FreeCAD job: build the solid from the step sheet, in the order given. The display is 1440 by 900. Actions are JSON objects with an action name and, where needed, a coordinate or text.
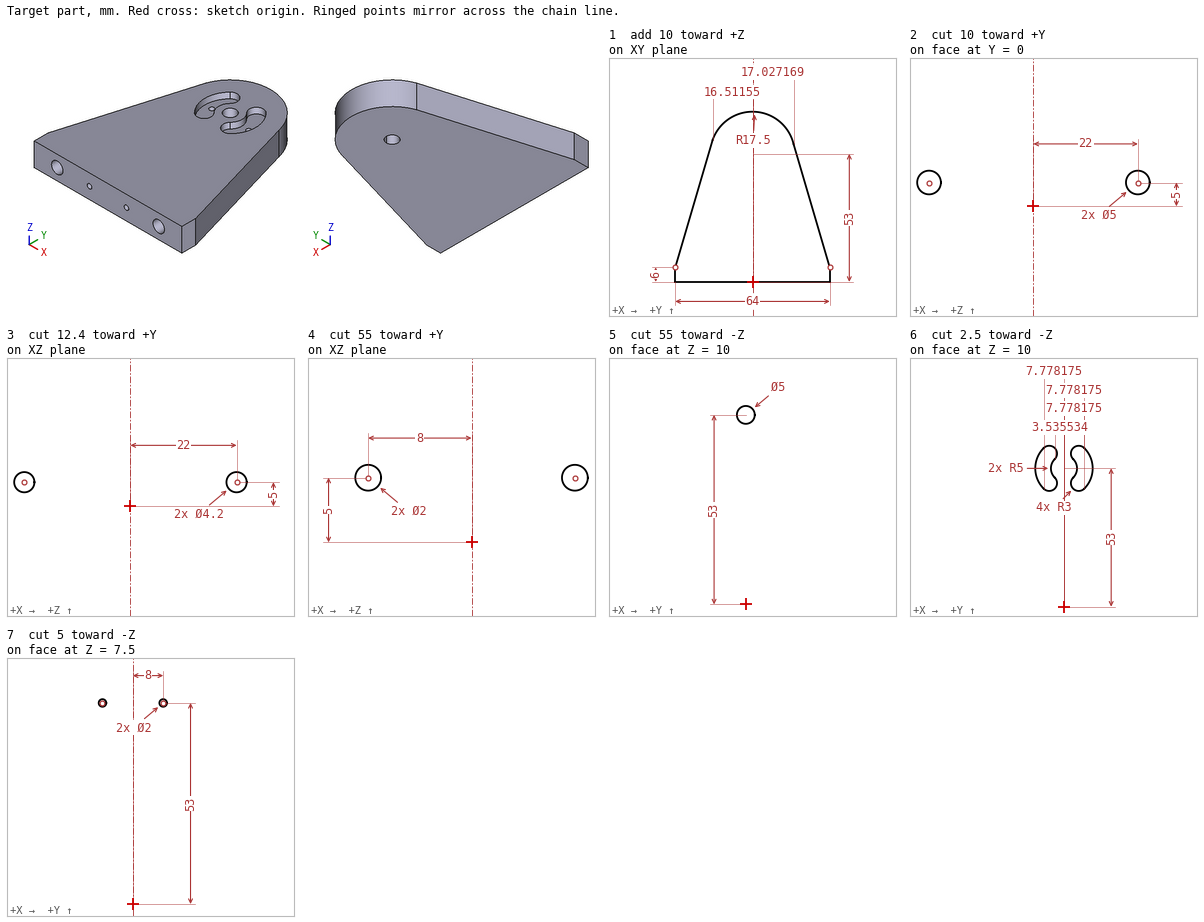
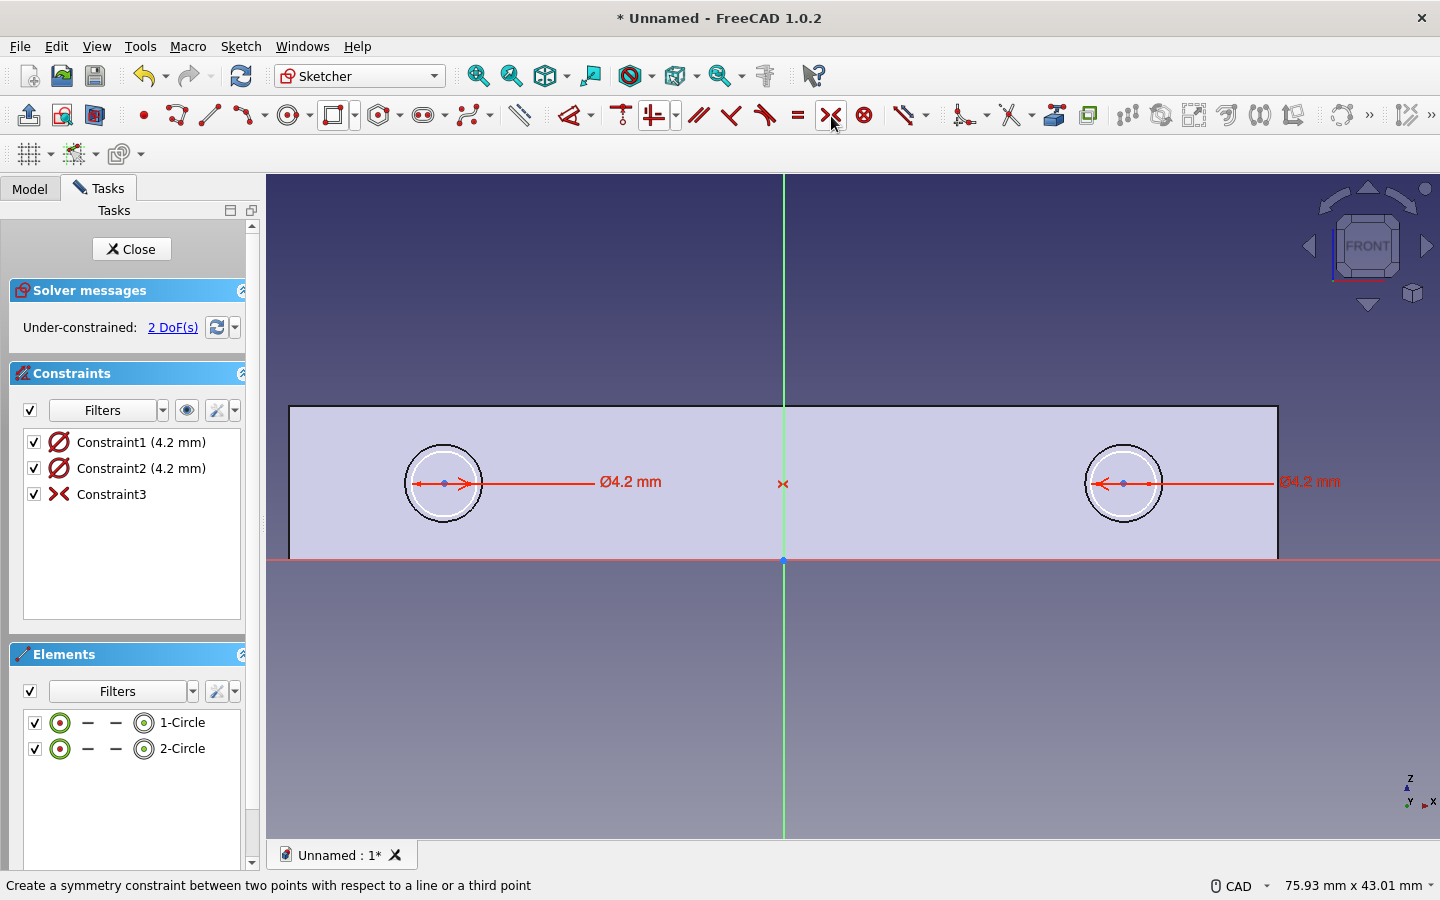
{"action": "left_click", "coordinate": [1123, 484]}
{"action": "left_click", "coordinate": [1157, 522]}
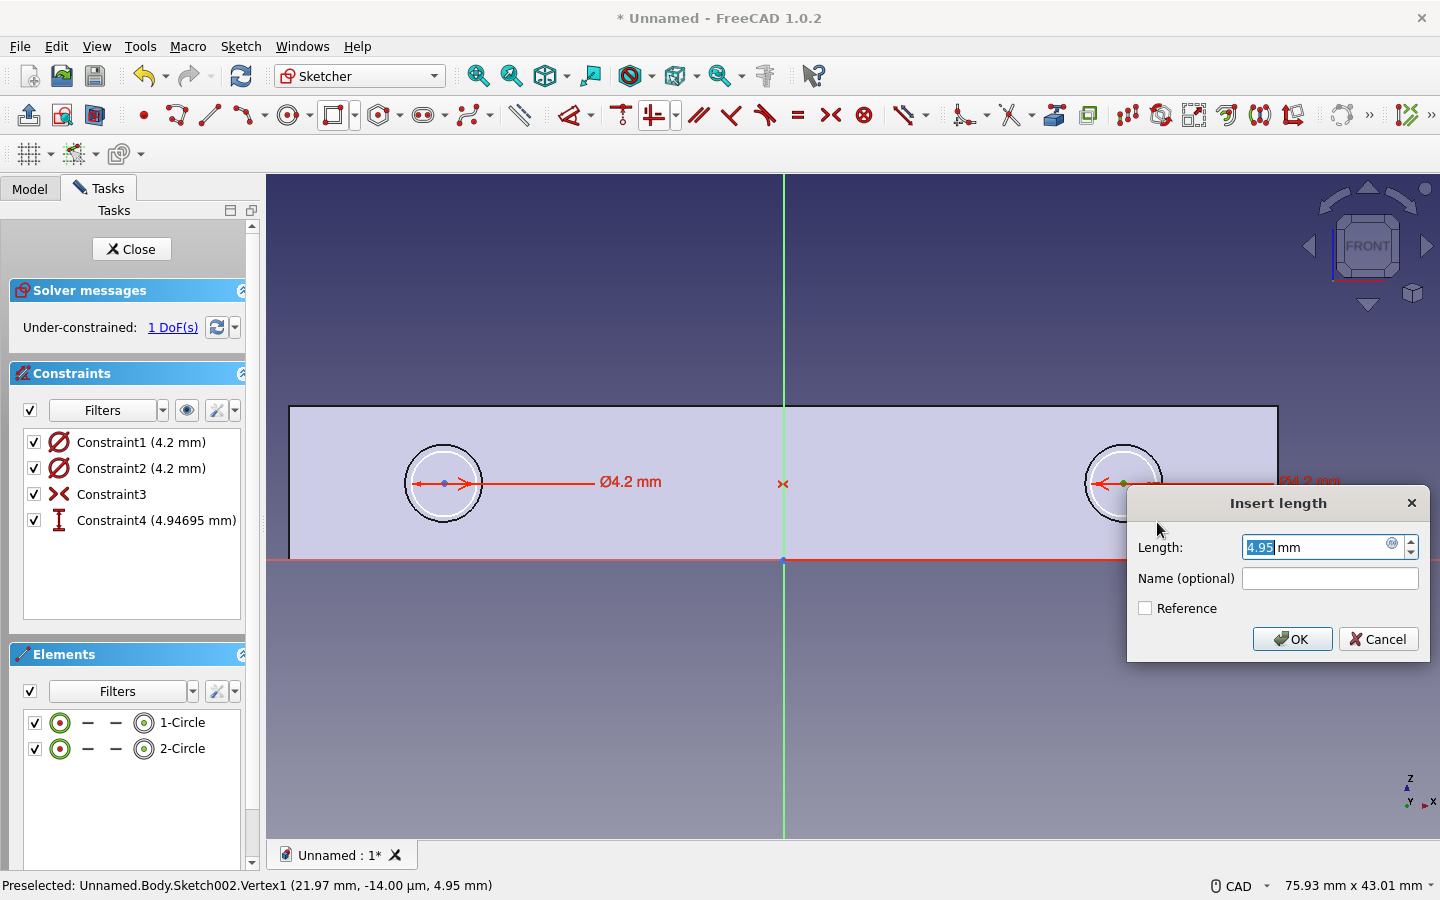
{"action": "type", "text": "5"}
{"action": "key", "text": "Return"}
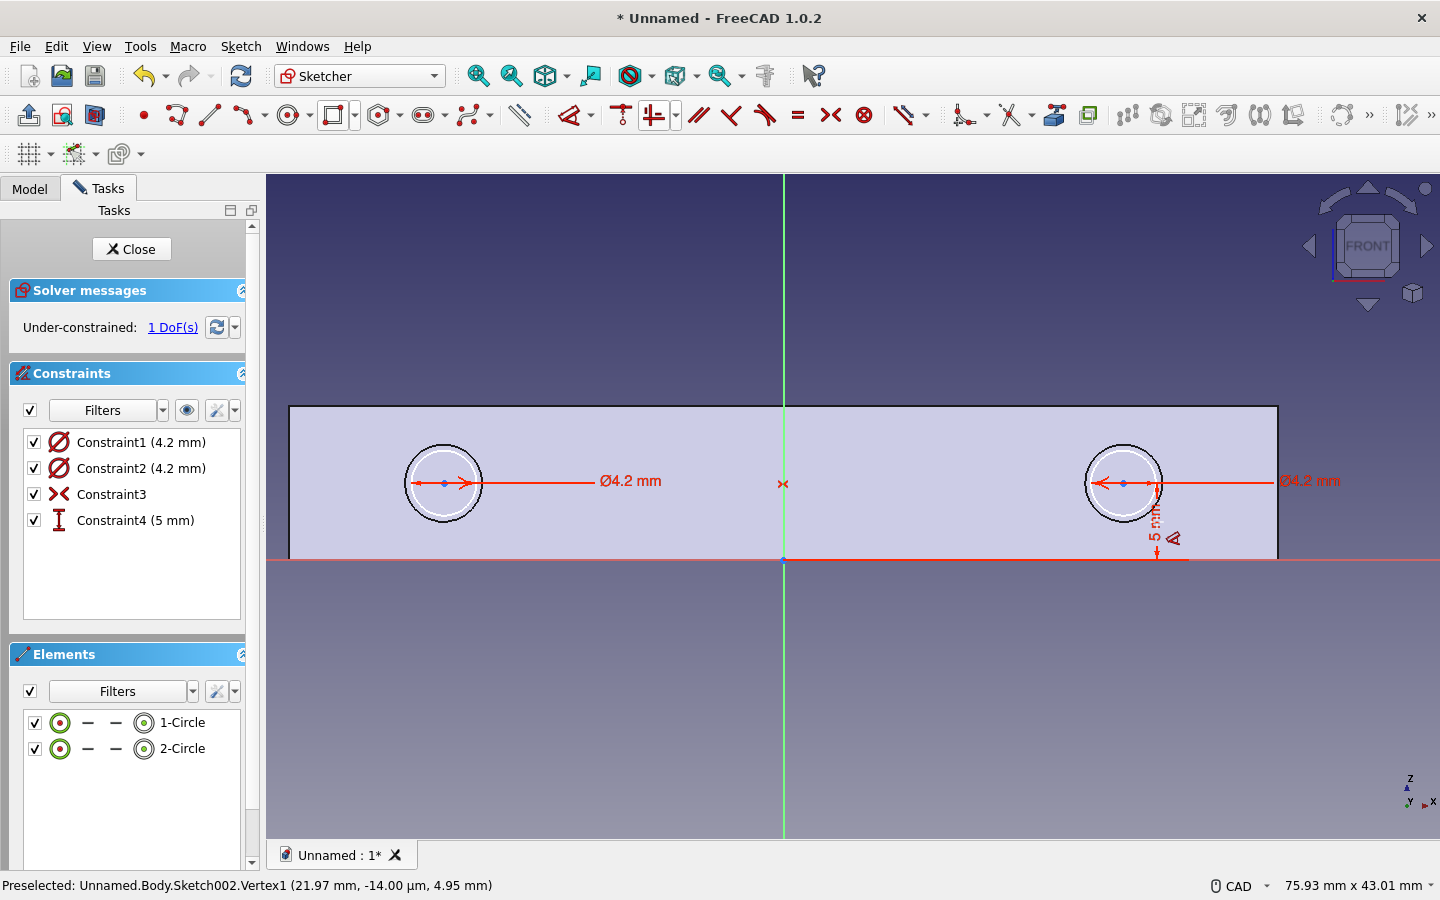
{"action": "left_click", "coordinate": [1123, 483]}
{"action": "left_click", "coordinate": [954, 594]}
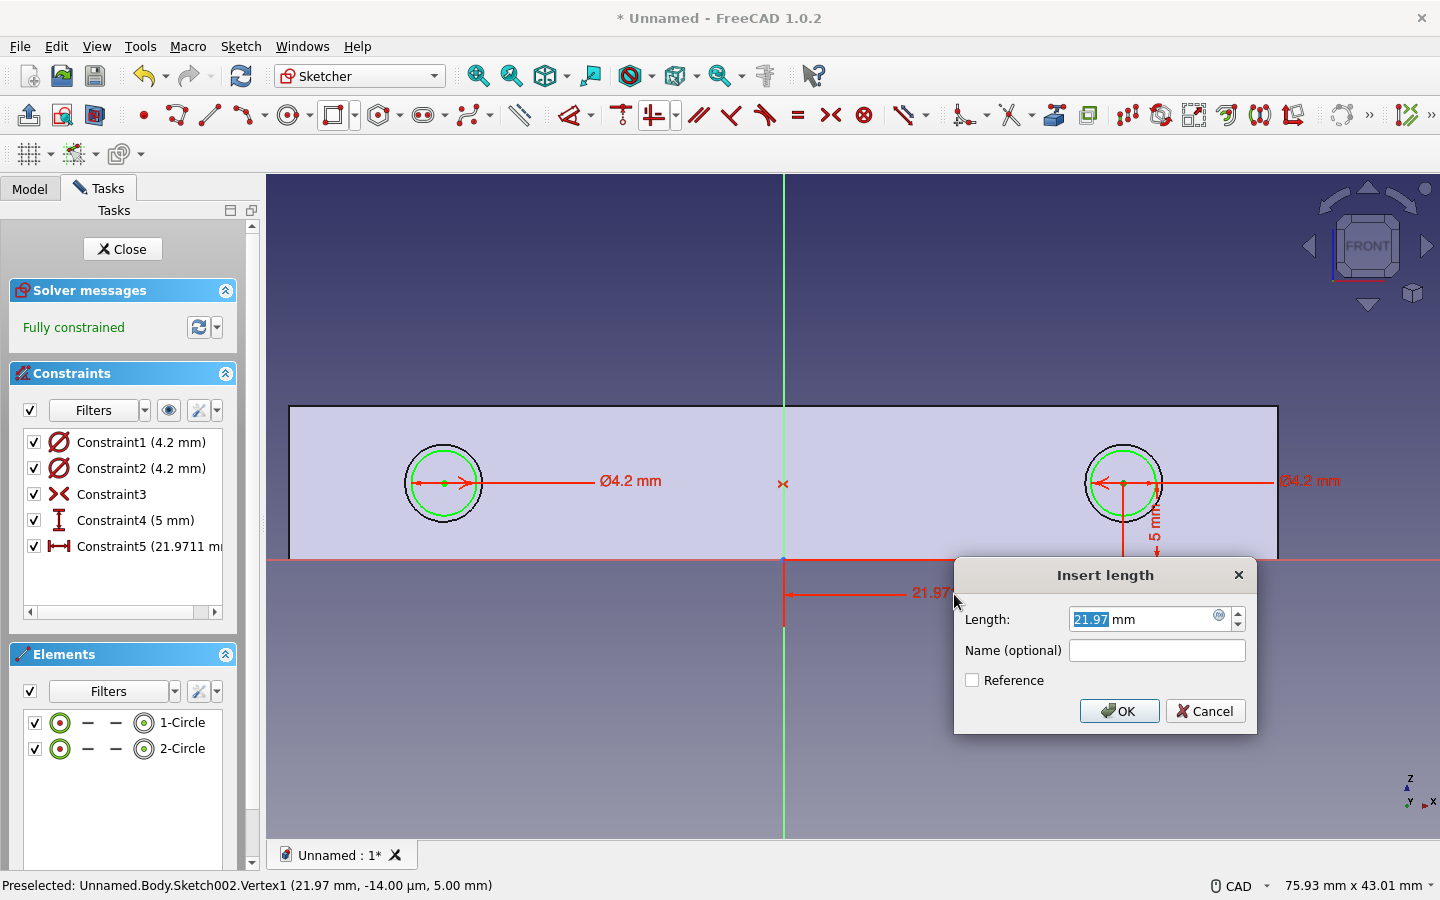
{"action": "type", "text": "22"}
{"action": "key", "text": "Return"}
{"action": "key", "text": "Escape"}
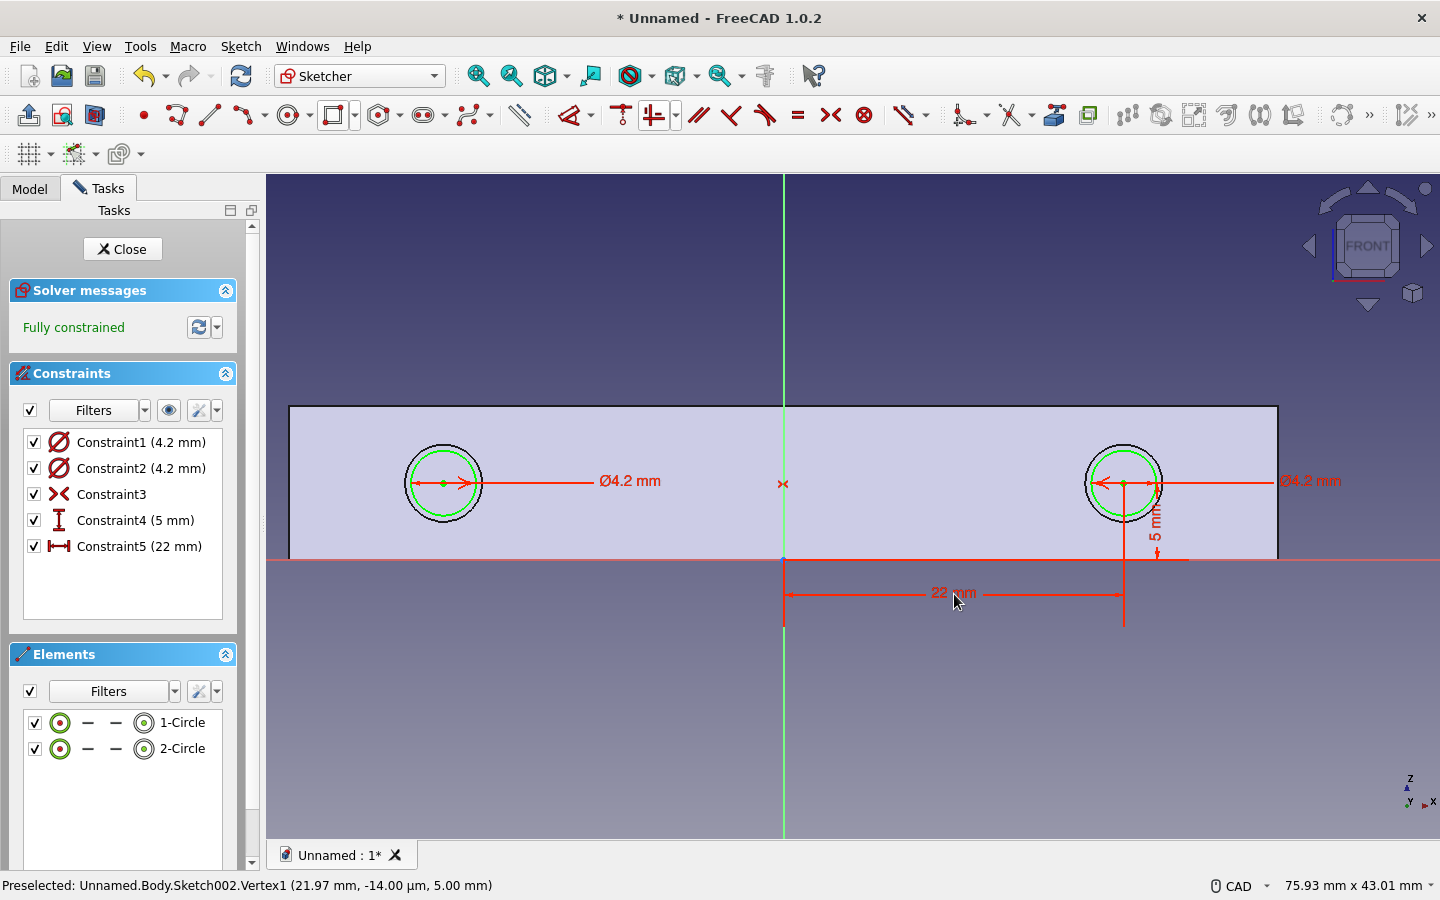
{"action": "left_click", "coordinate": [123, 249]}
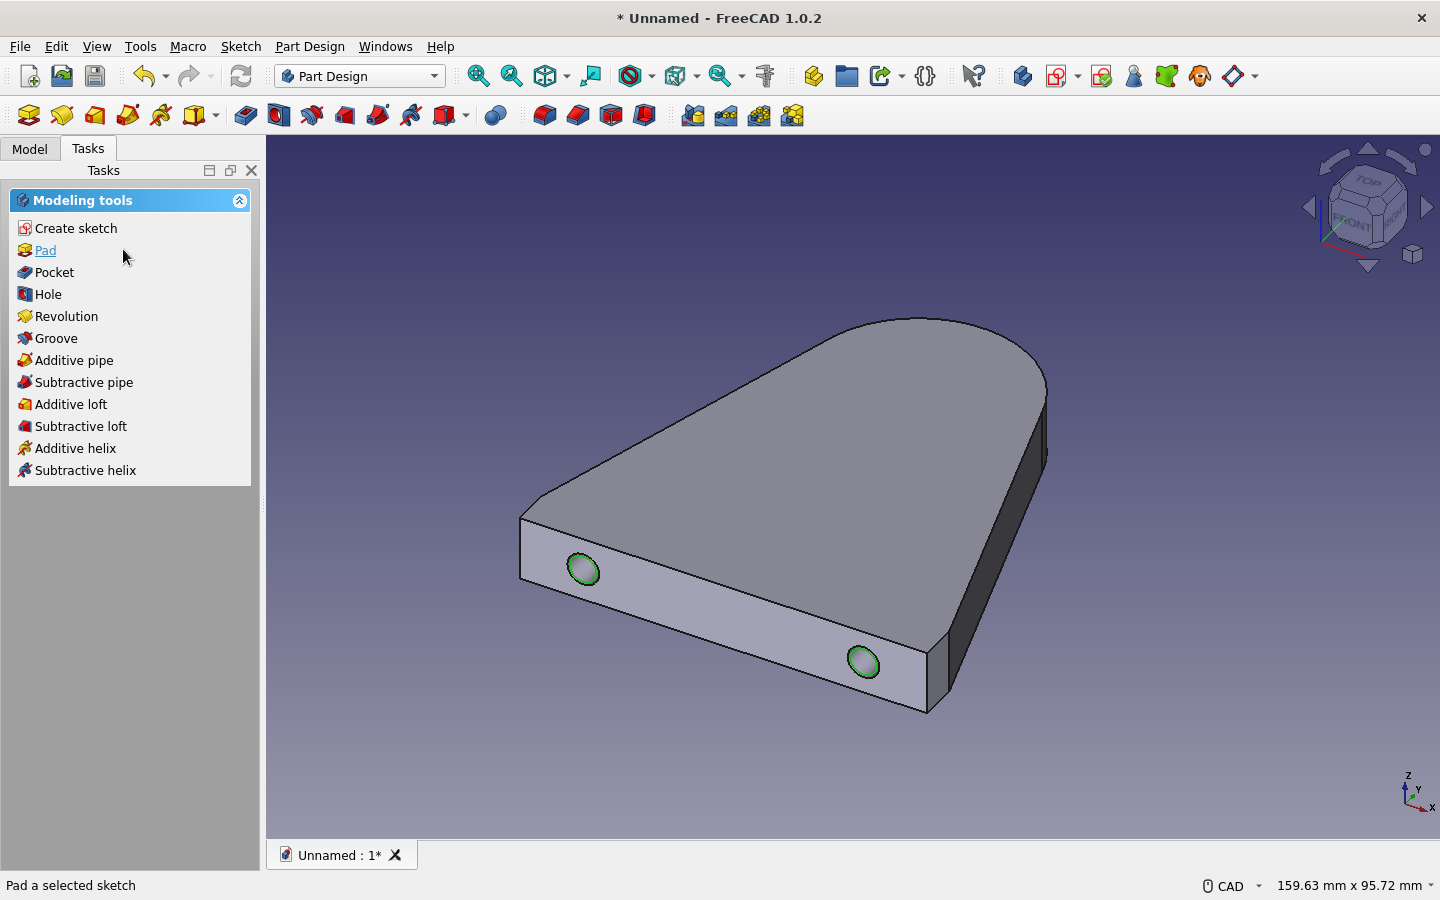
{"action": "left_click", "coordinate": [246, 116]}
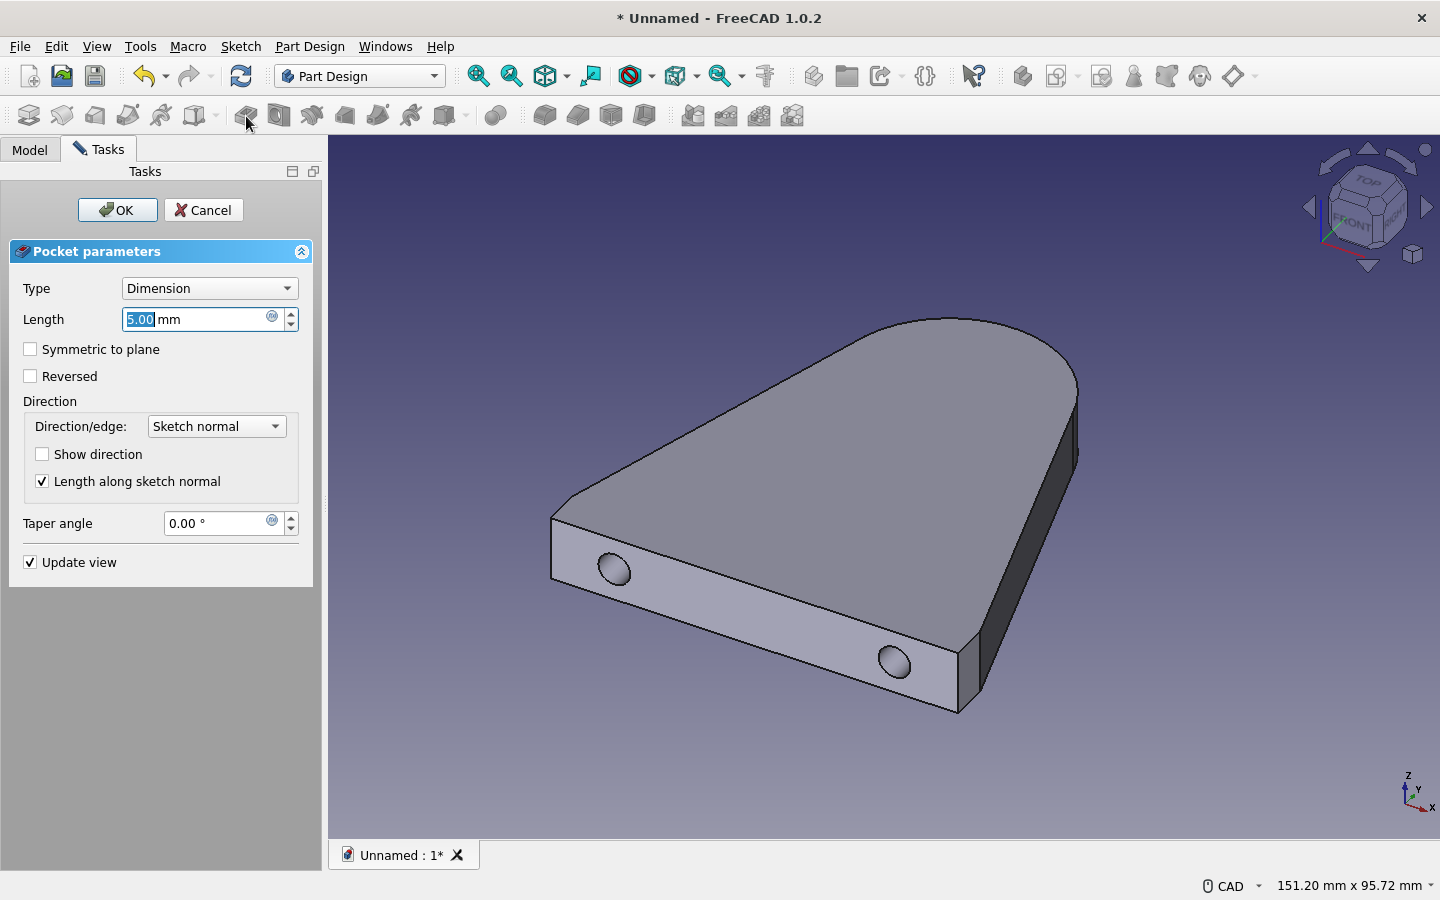
{"action": "type", "text": "12.4"}
{"action": "key", "text": "Tab"}